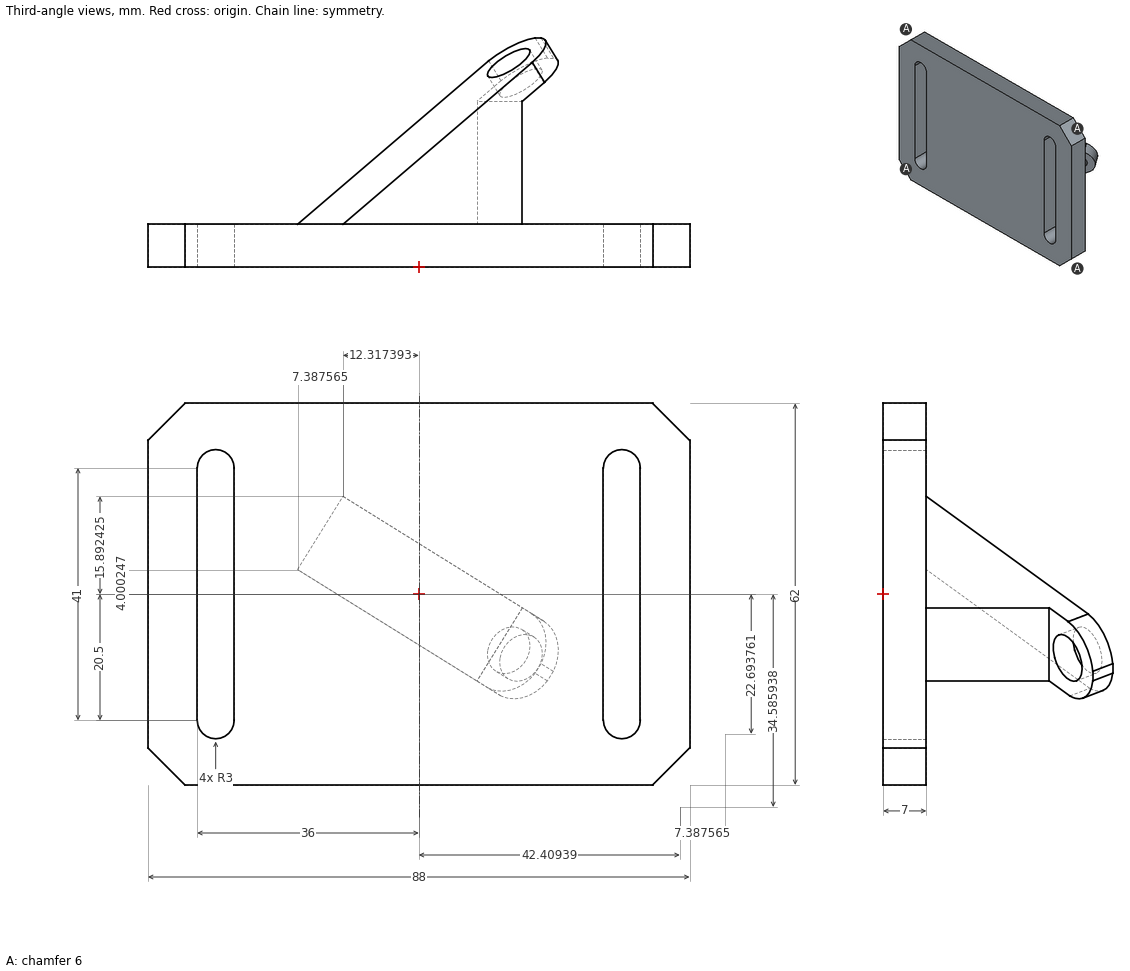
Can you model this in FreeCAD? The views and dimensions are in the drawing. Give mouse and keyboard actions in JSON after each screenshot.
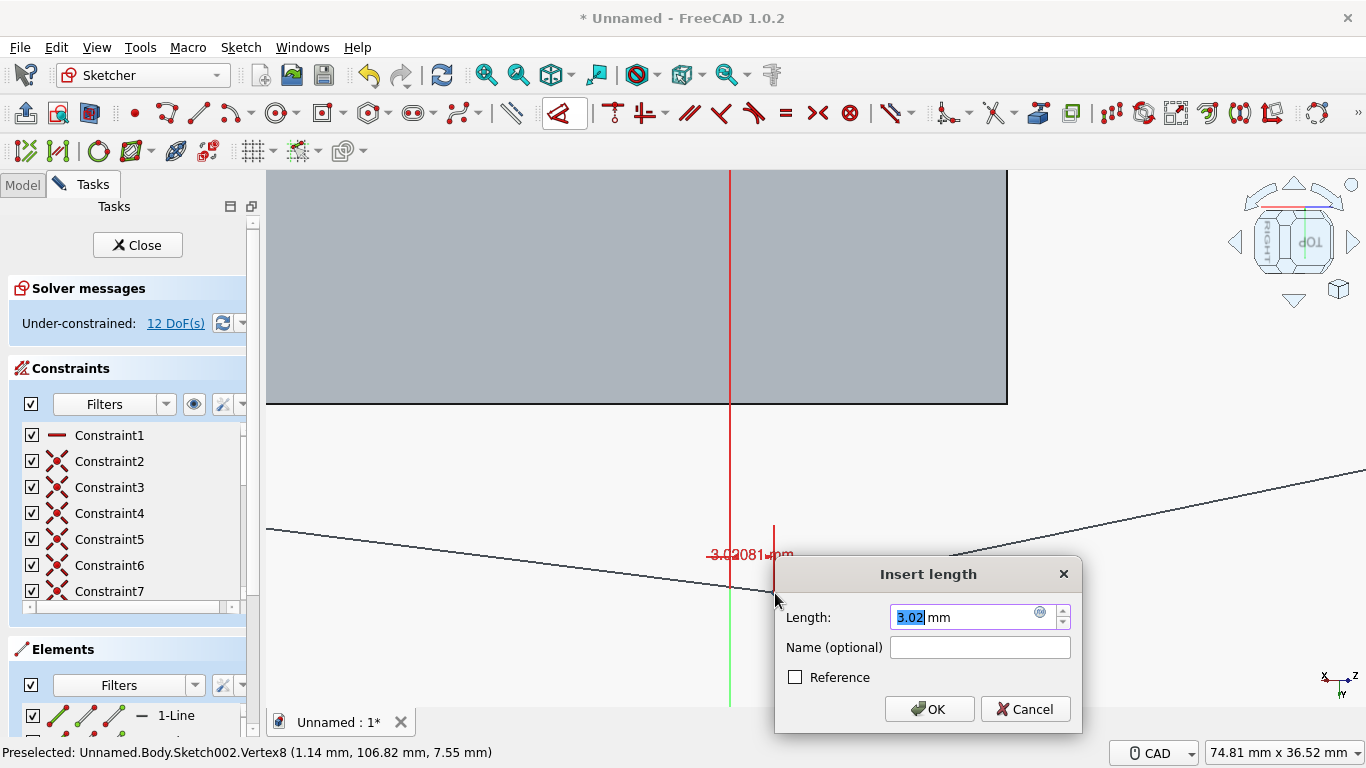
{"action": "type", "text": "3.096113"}
{"action": "key", "text": "Return"}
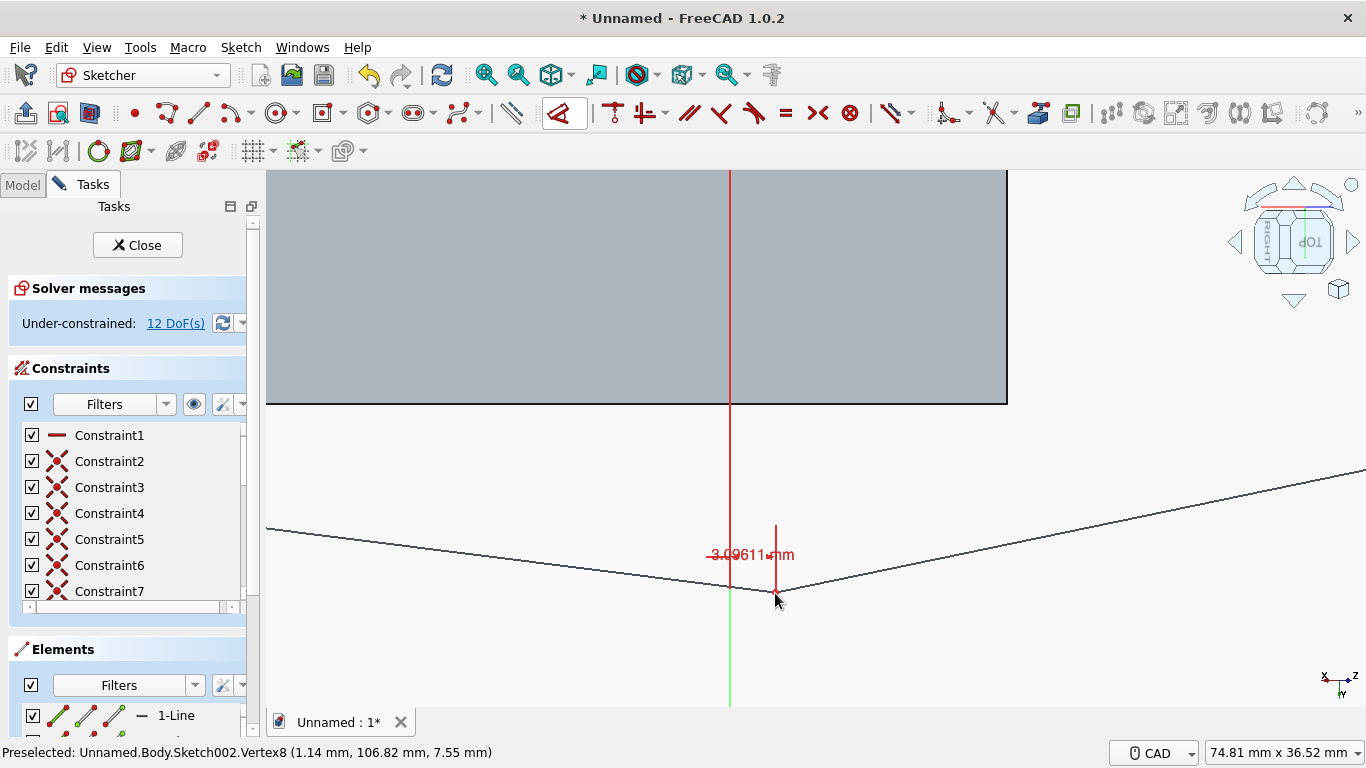
{"action": "scroll", "coordinate": [777, 598], "scroll_direction": "down", "scroll_amount": 8}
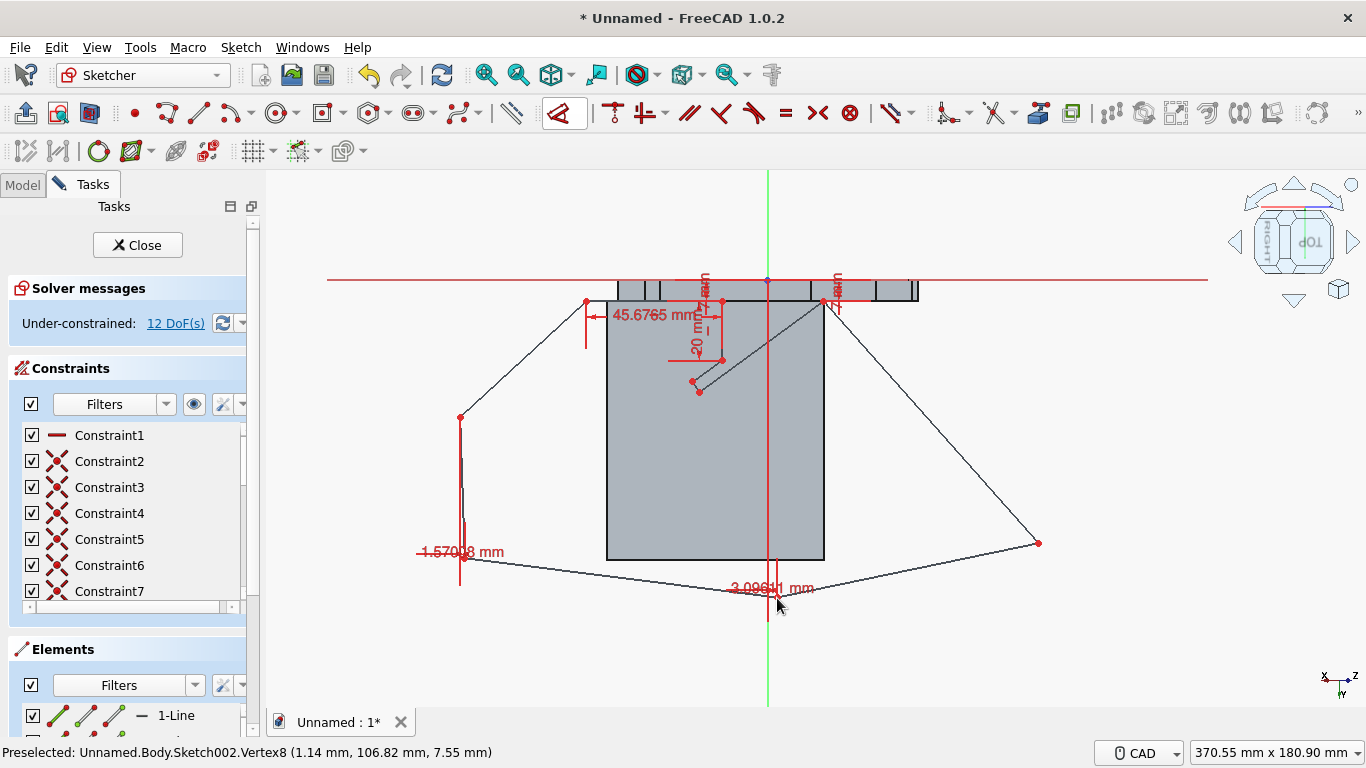
{"action": "scroll", "coordinate": [698, 389], "scroll_direction": "up", "scroll_amount": 9}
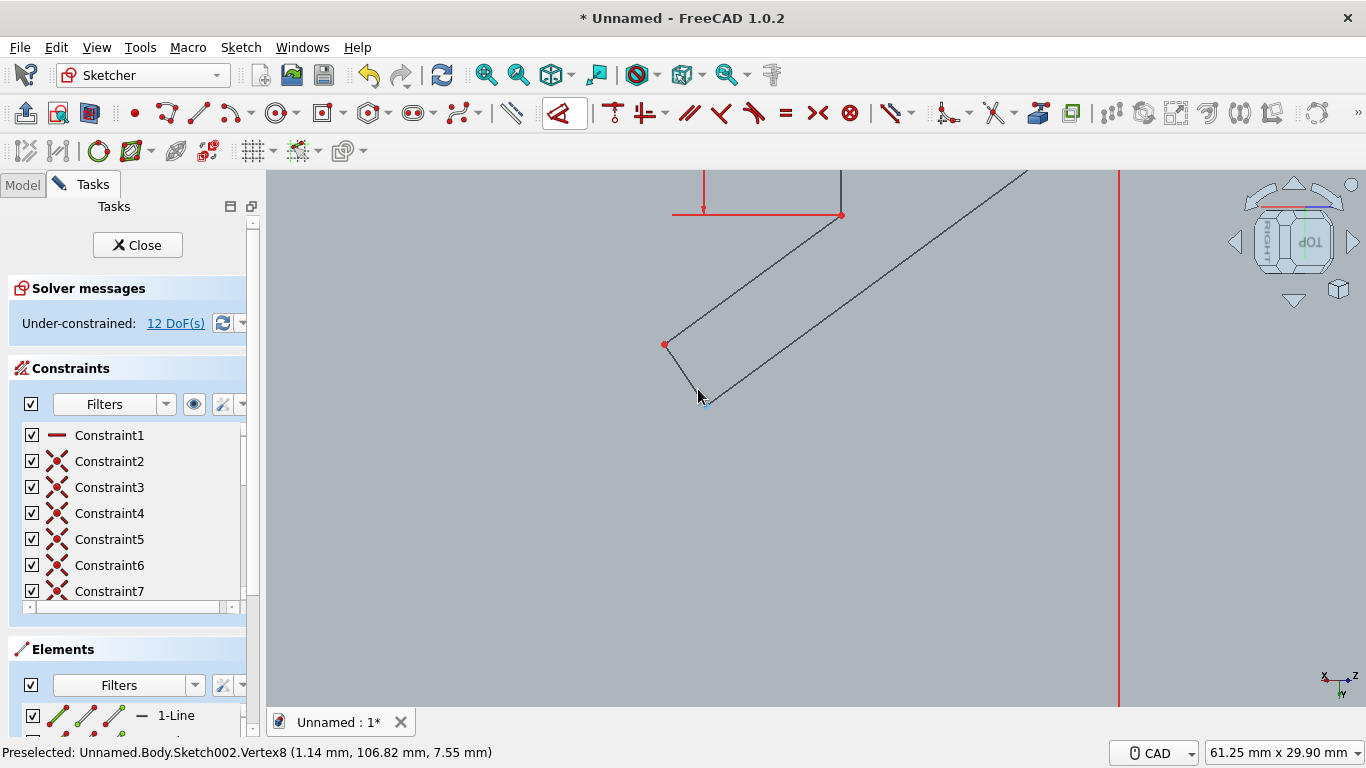
{"action": "left_click", "coordinate": [694, 388]}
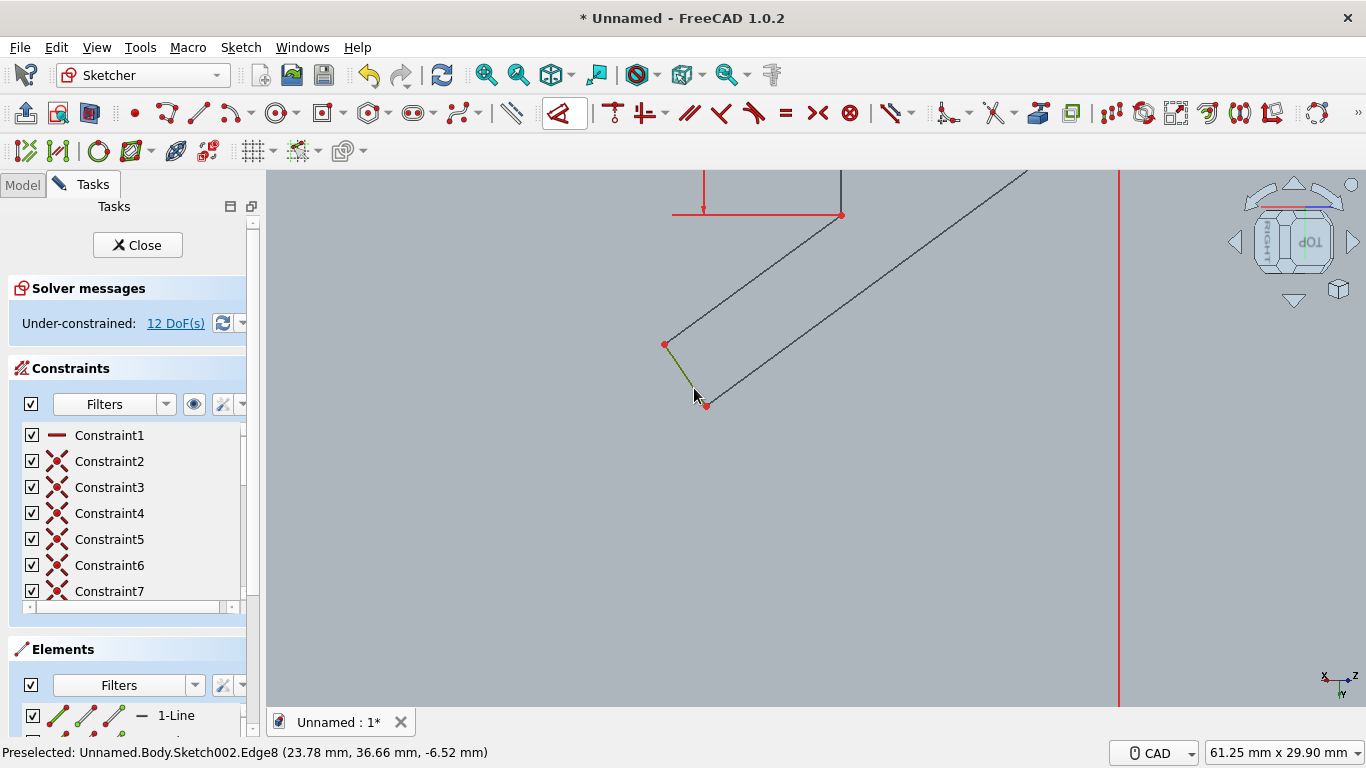
{"action": "left_click", "coordinate": [582, 114]}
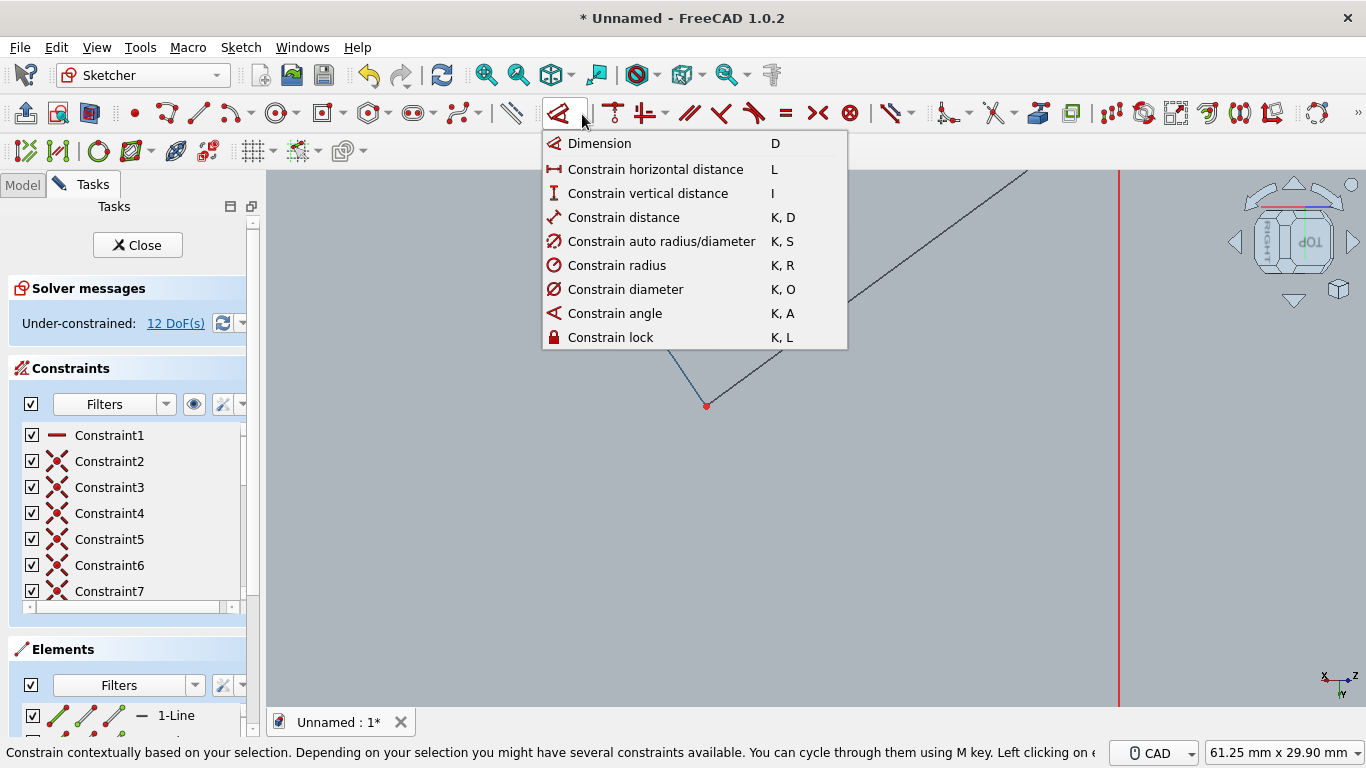
{"action": "left_click", "coordinate": [695, 169]}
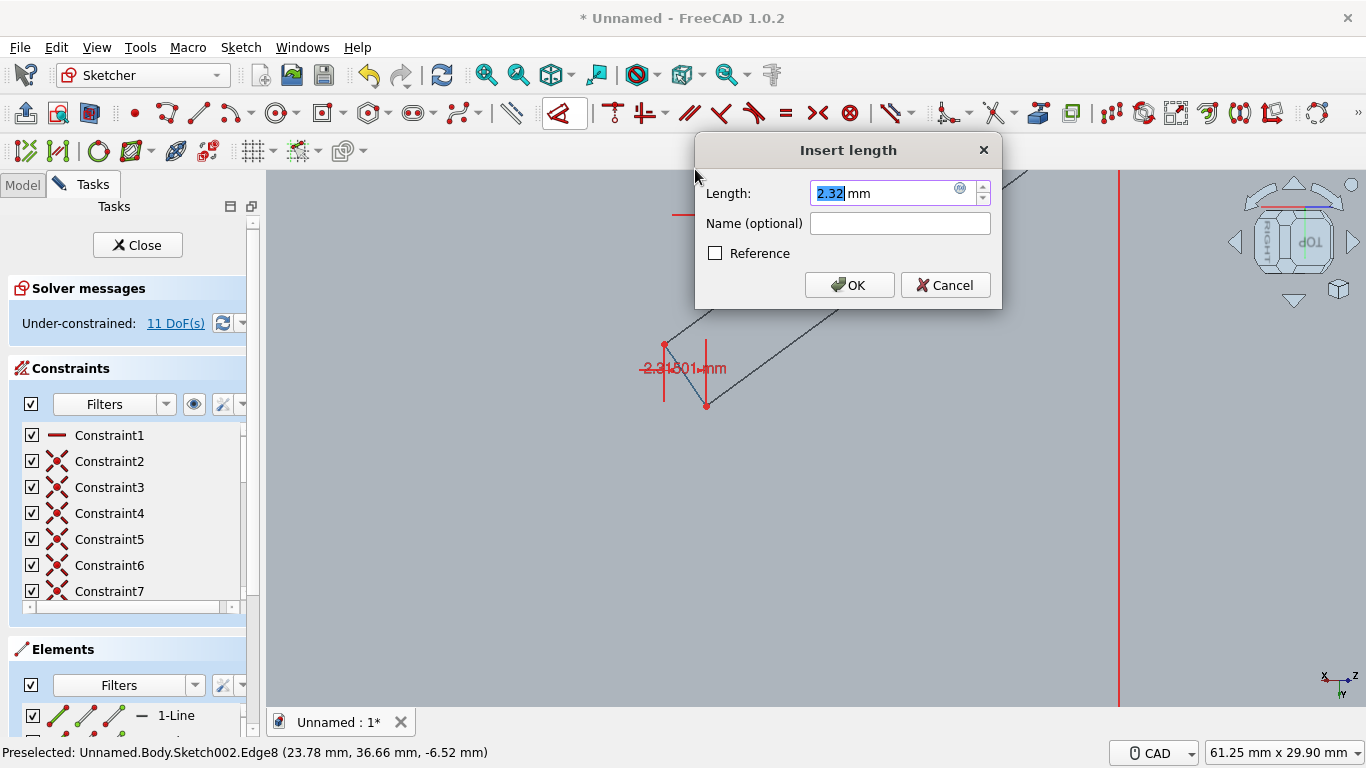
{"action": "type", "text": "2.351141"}
{"action": "key", "text": "Return"}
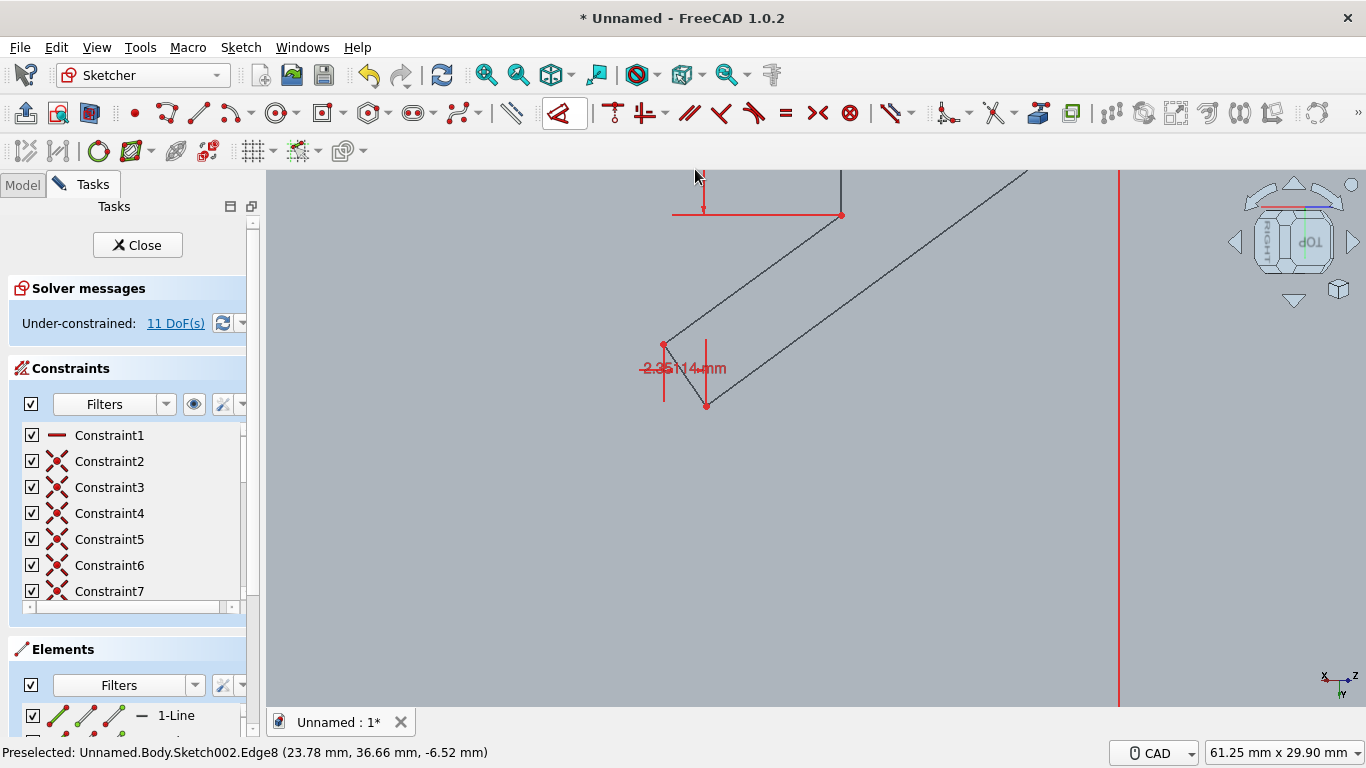
{"action": "left_click", "coordinate": [693, 388]}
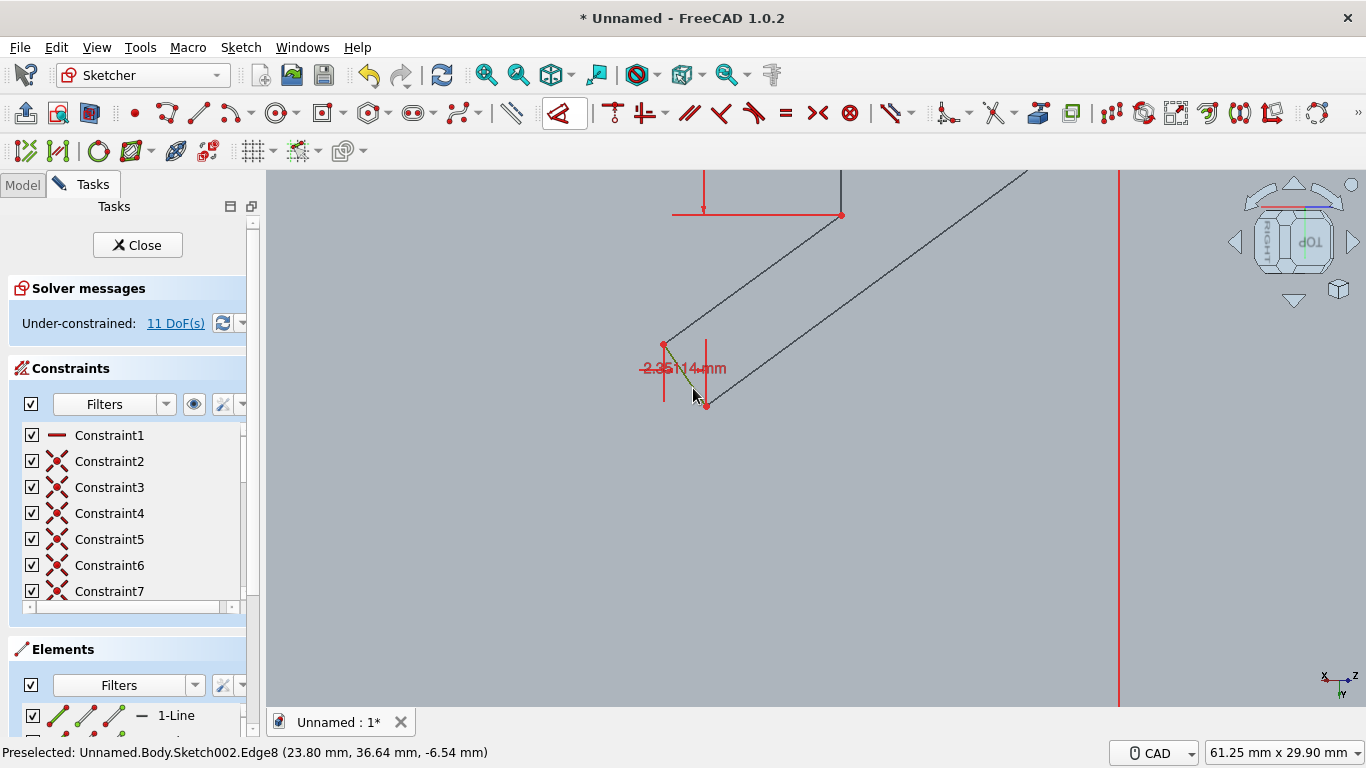
{"action": "left_click", "coordinate": [582, 114]}